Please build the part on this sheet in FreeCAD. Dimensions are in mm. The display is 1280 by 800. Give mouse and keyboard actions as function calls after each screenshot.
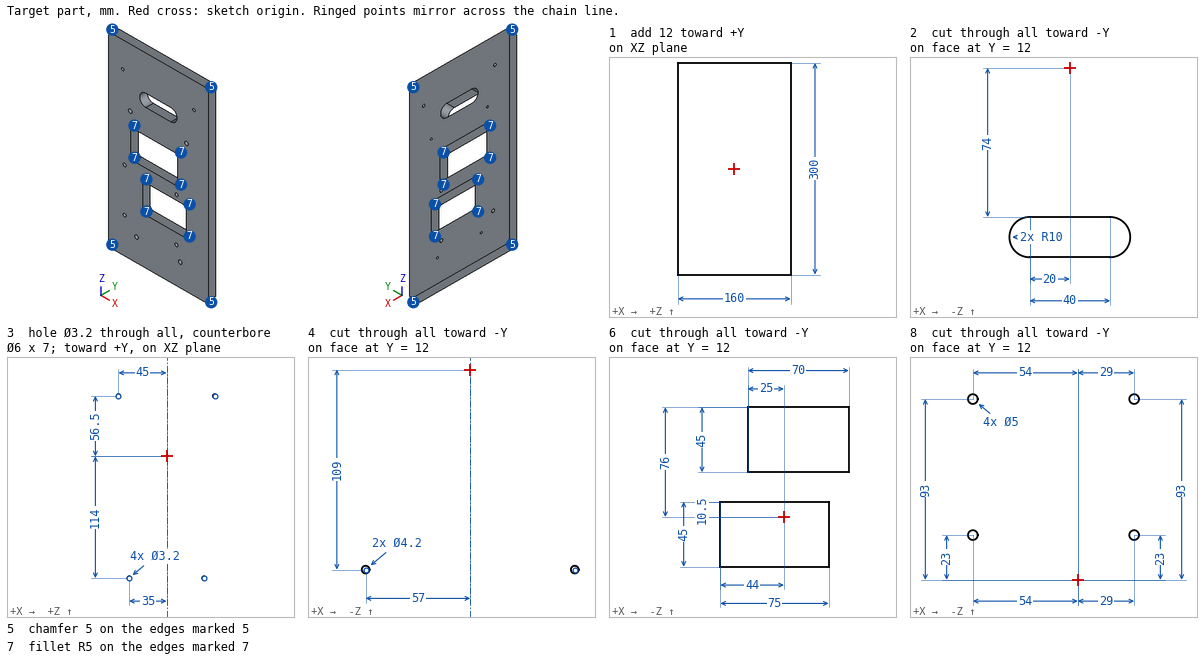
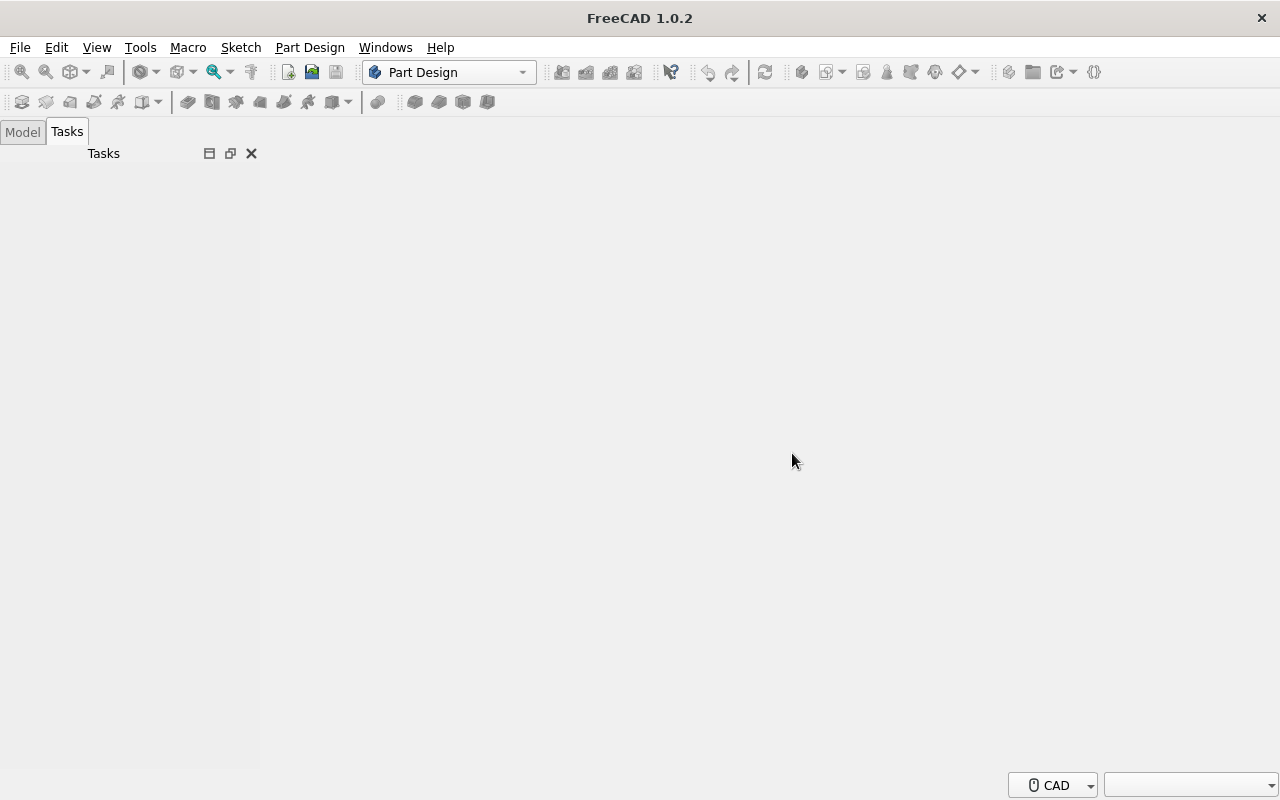
click(288, 72)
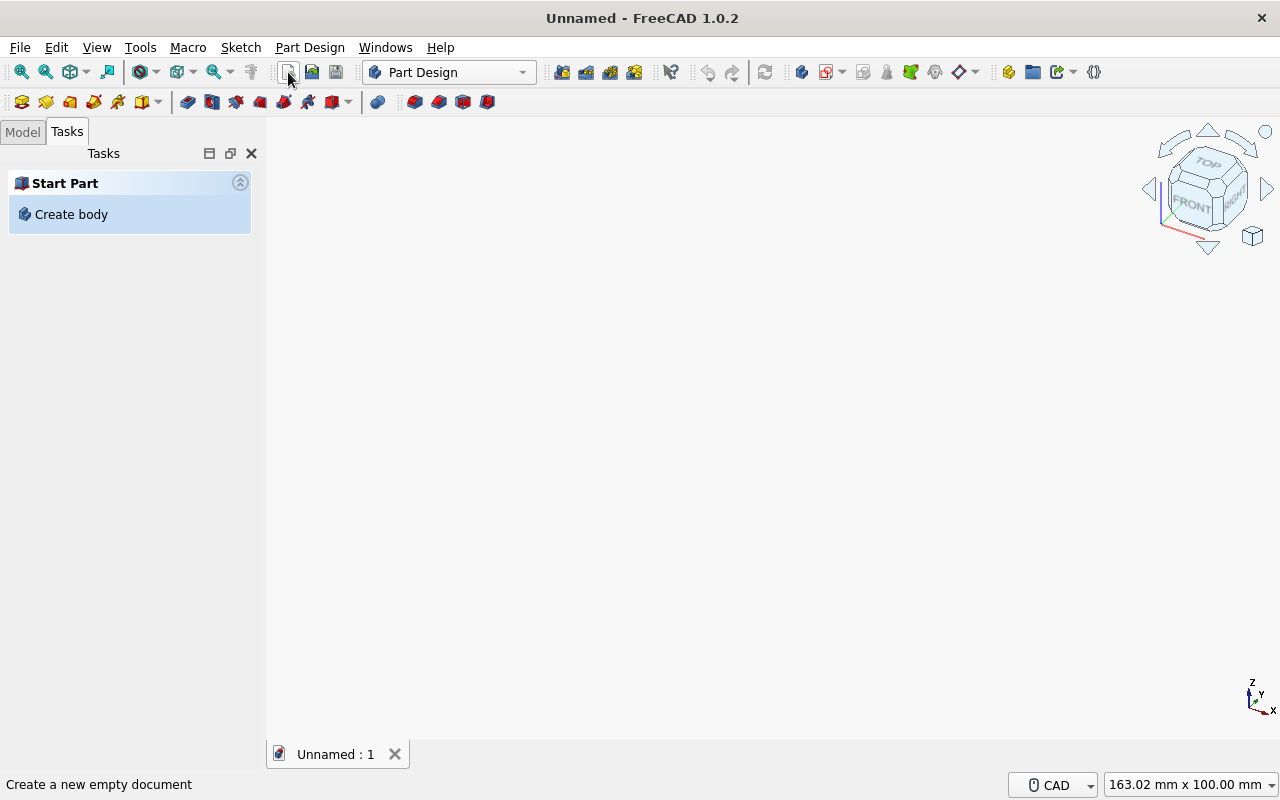
click(826, 72)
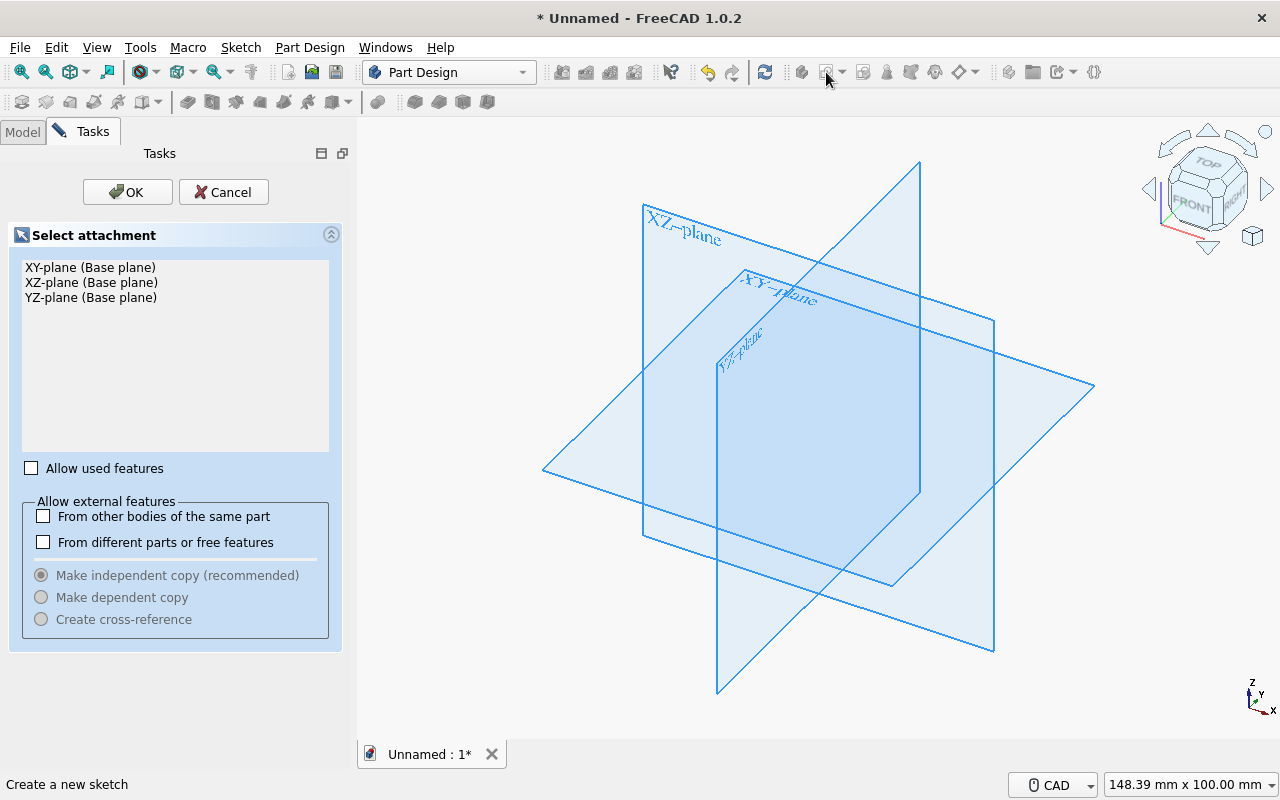
click(82, 282)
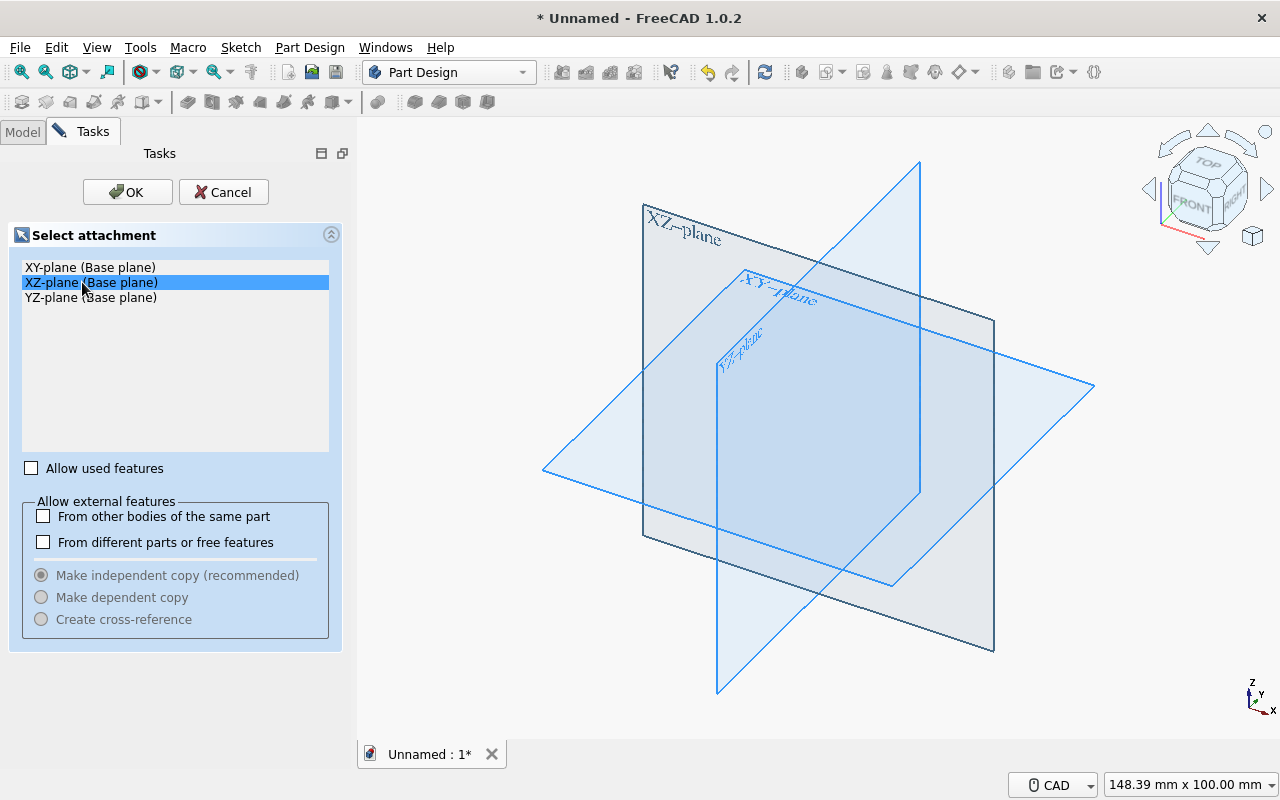
click(128, 192)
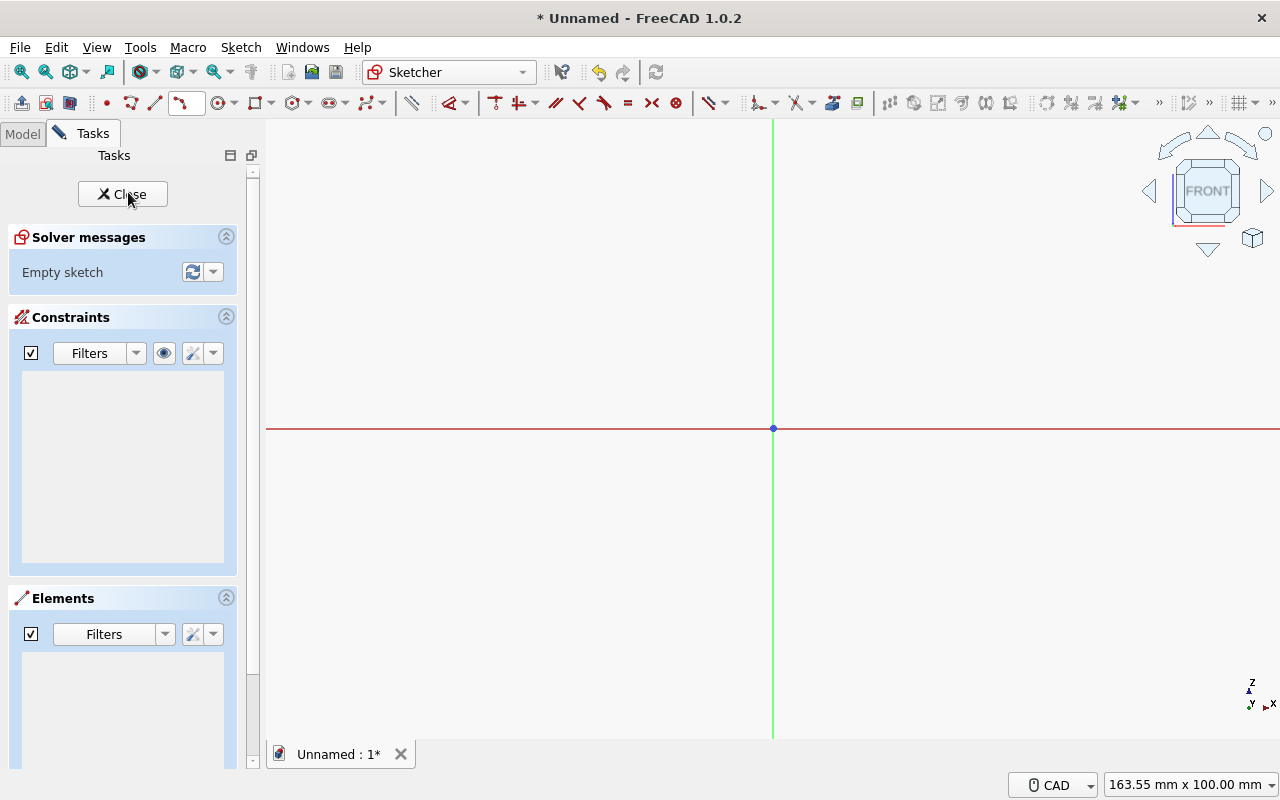
scroll(687, 429, down, 8)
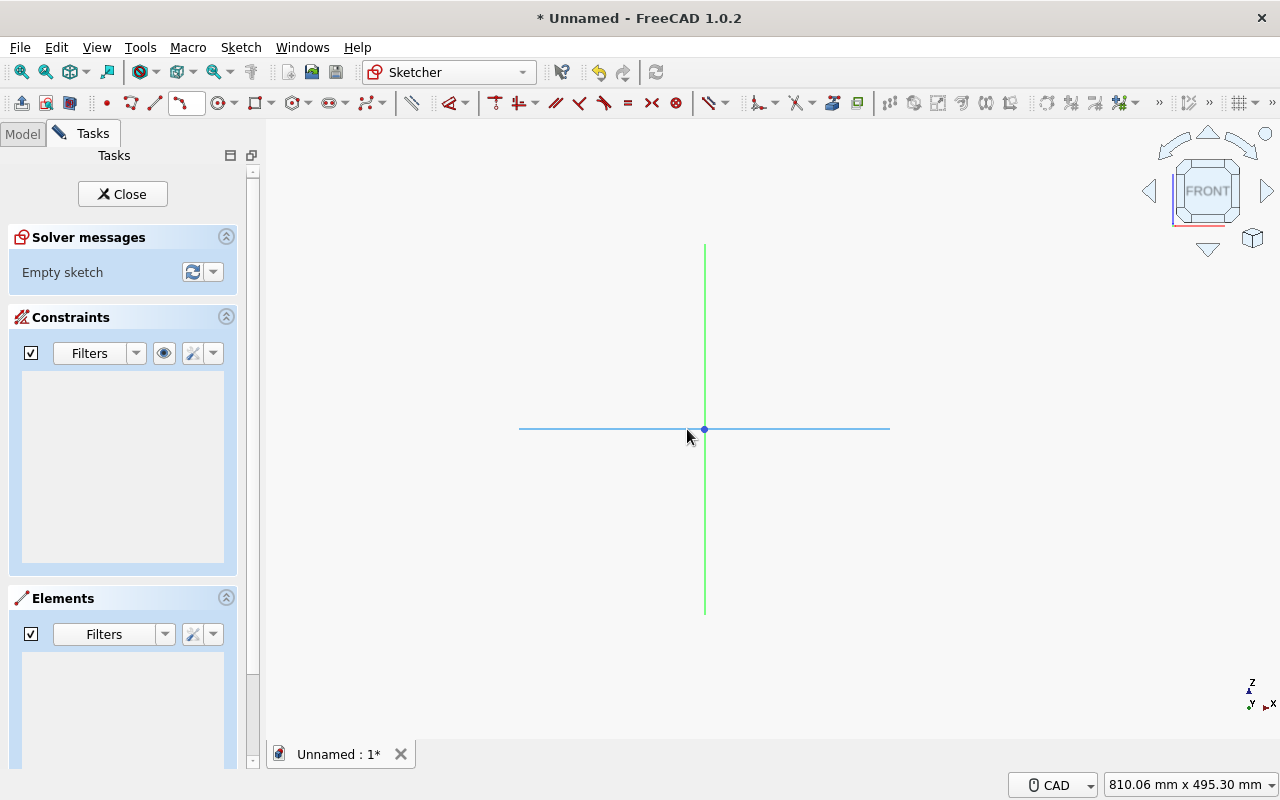
click(274, 104)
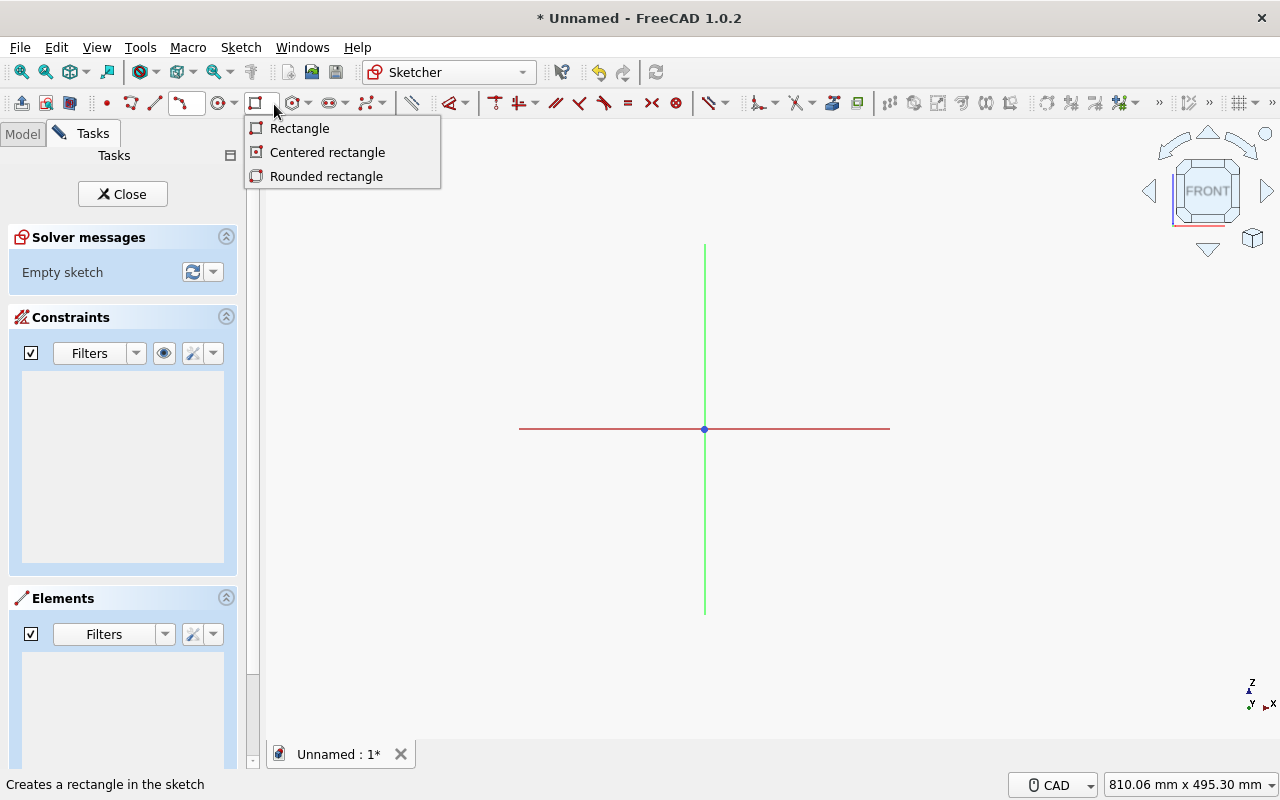
click(342, 152)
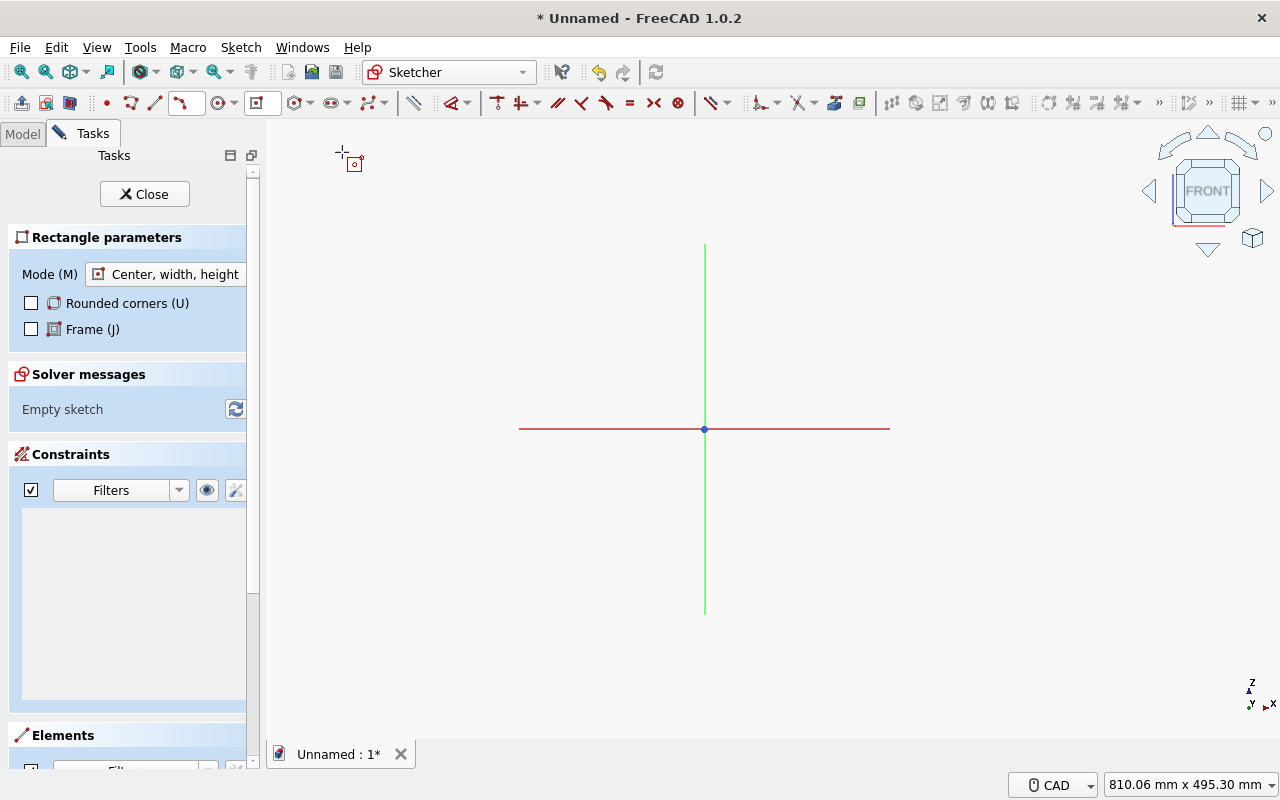
click(705, 429)
click(805, 242)
key(Escape)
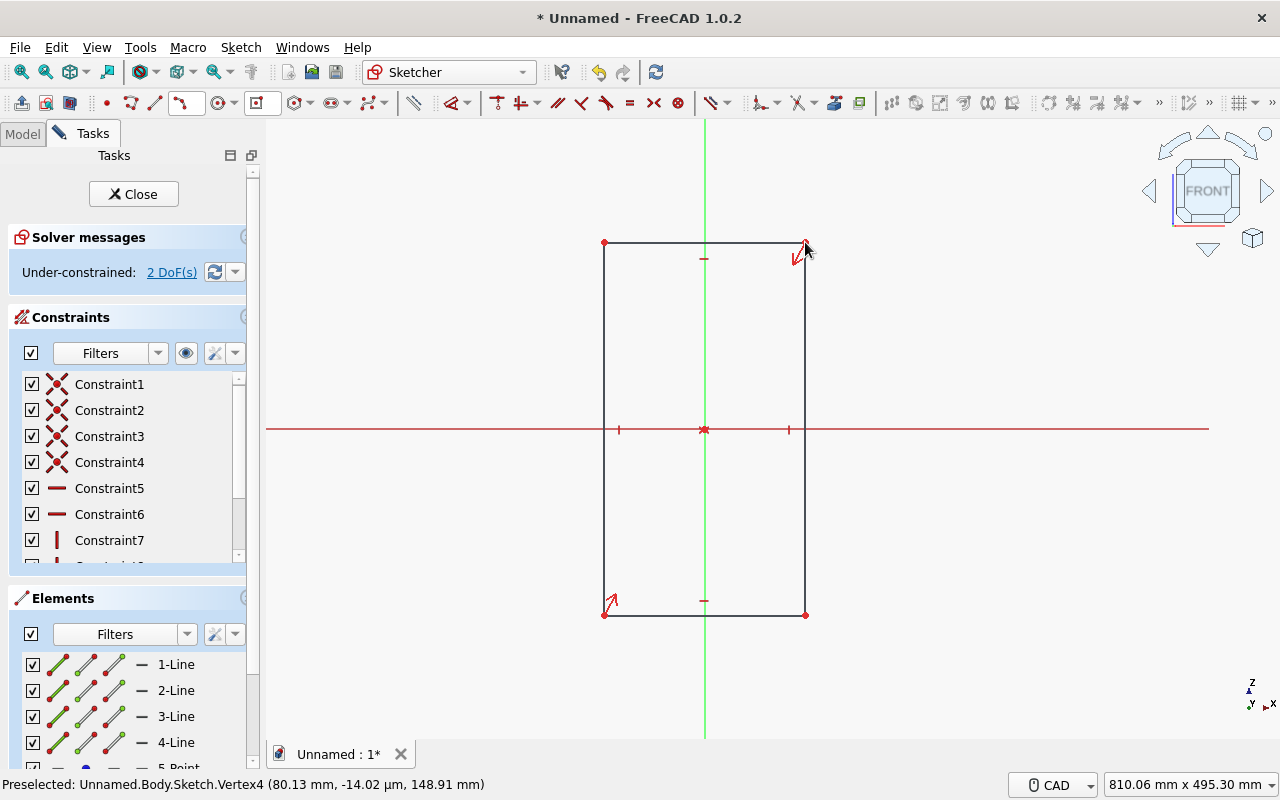
click(452, 104)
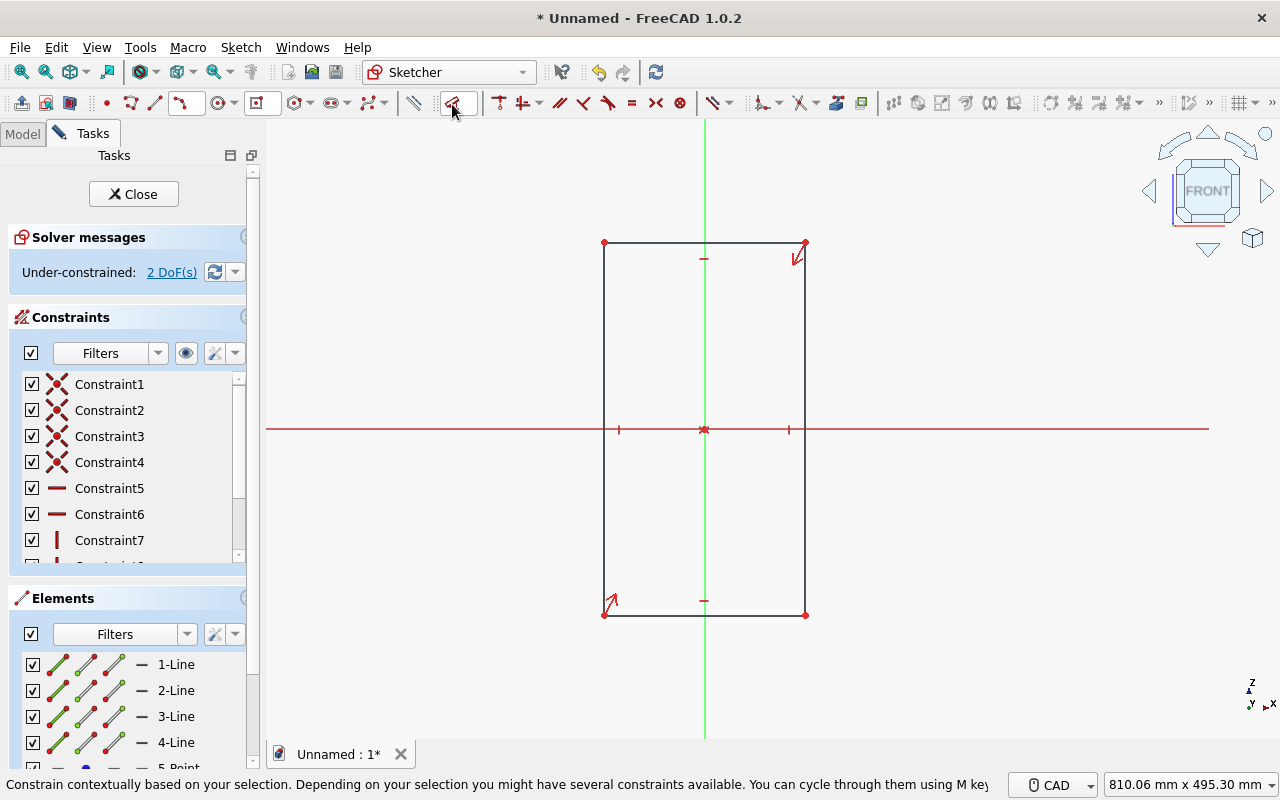
click(665, 616)
click(659, 650)